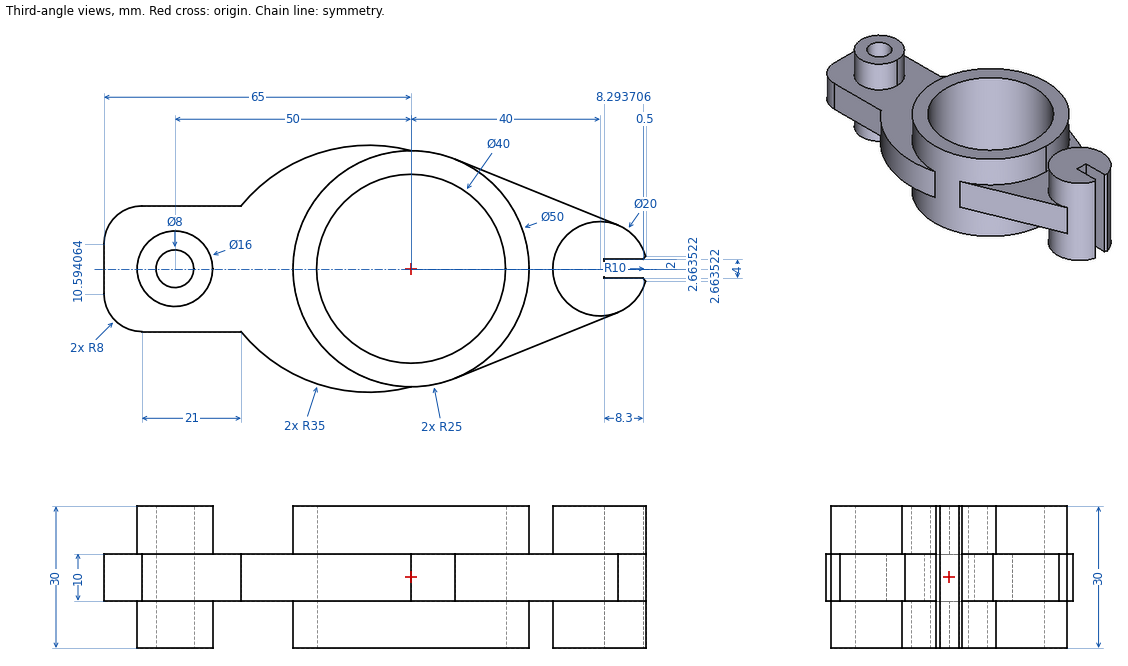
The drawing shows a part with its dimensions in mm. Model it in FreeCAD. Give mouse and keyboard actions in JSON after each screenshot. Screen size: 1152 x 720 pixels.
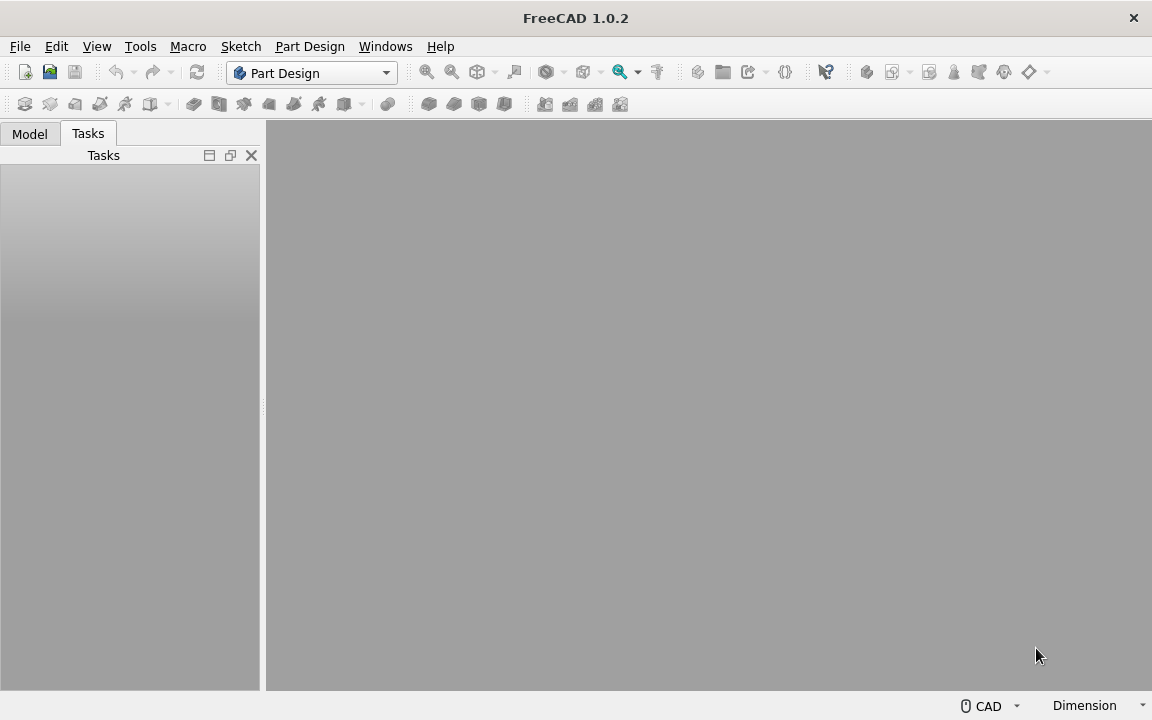
{"action": "left_click", "coordinate": [25, 72]}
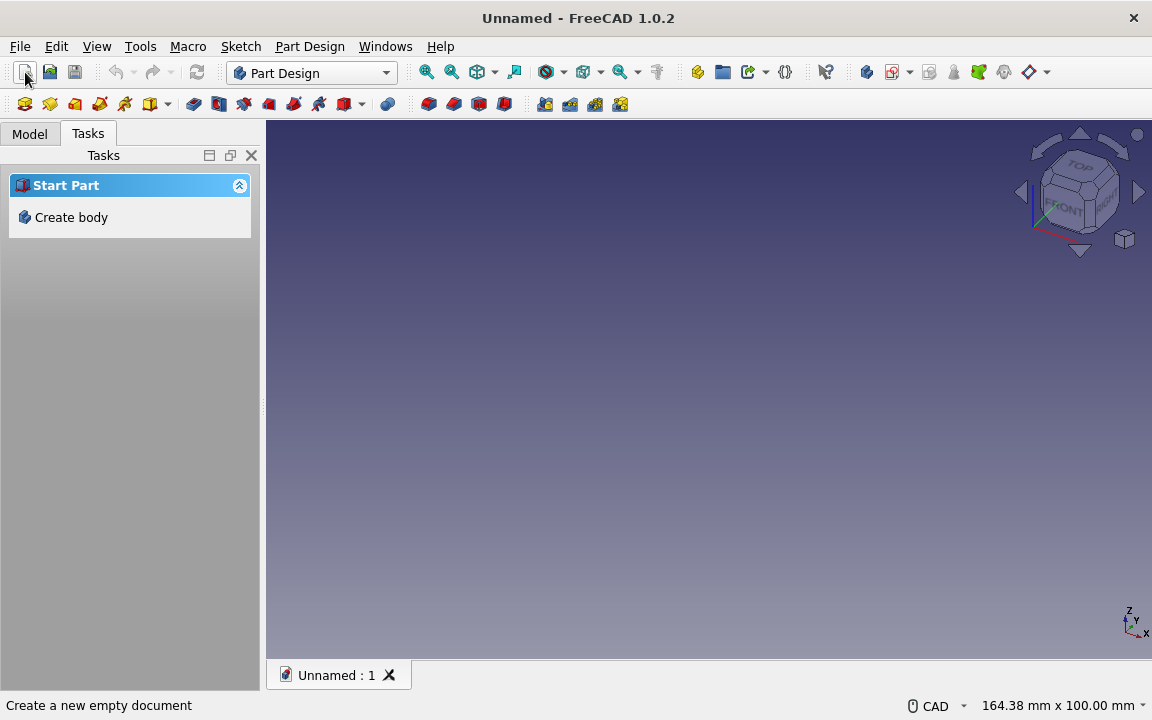
{"action": "left_click", "coordinate": [892, 72]}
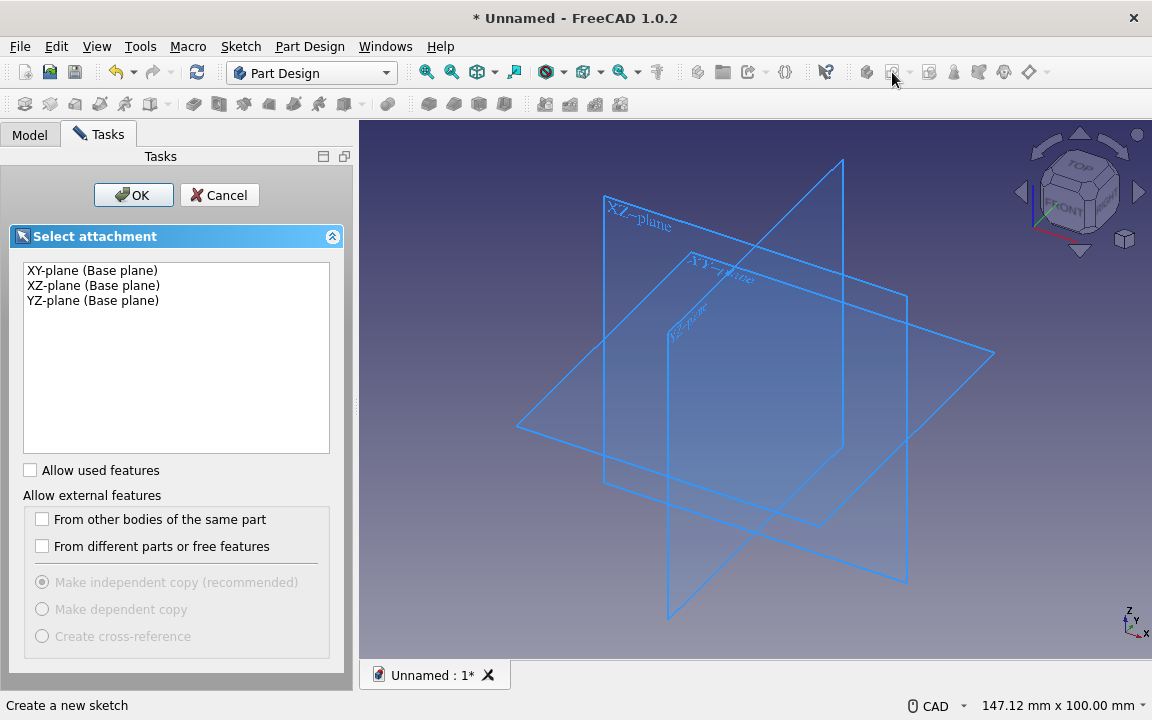
{"action": "left_click", "coordinate": [84, 270]}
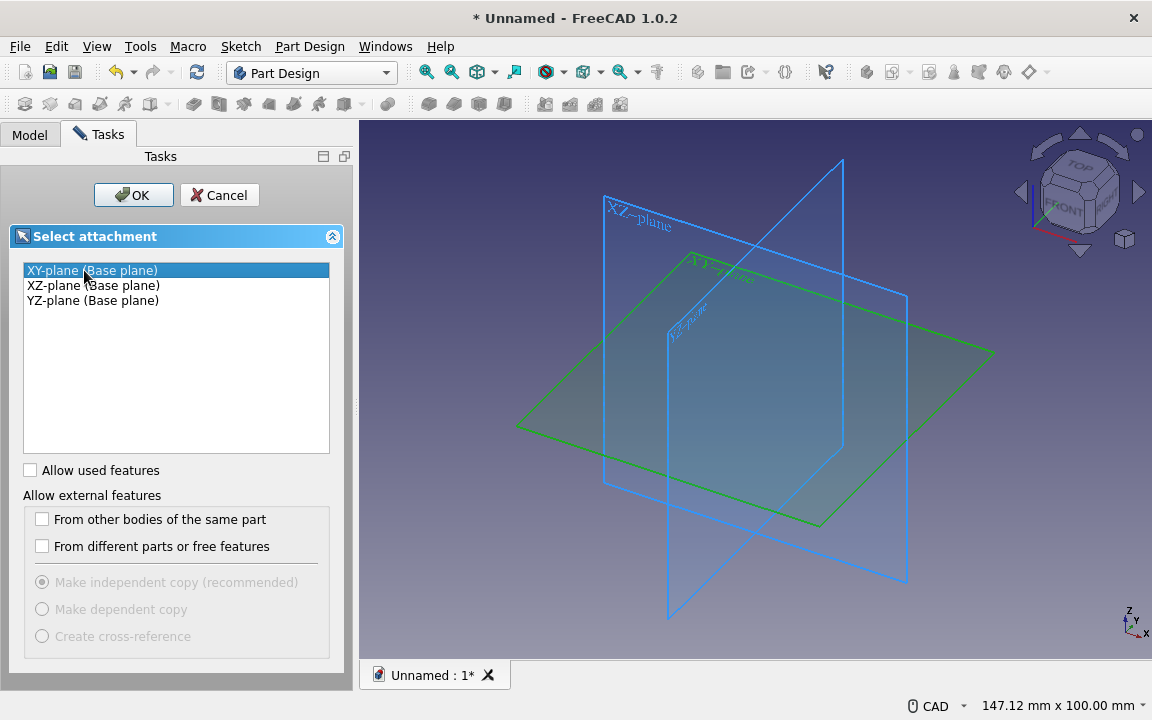
{"action": "left_click", "coordinate": [134, 195]}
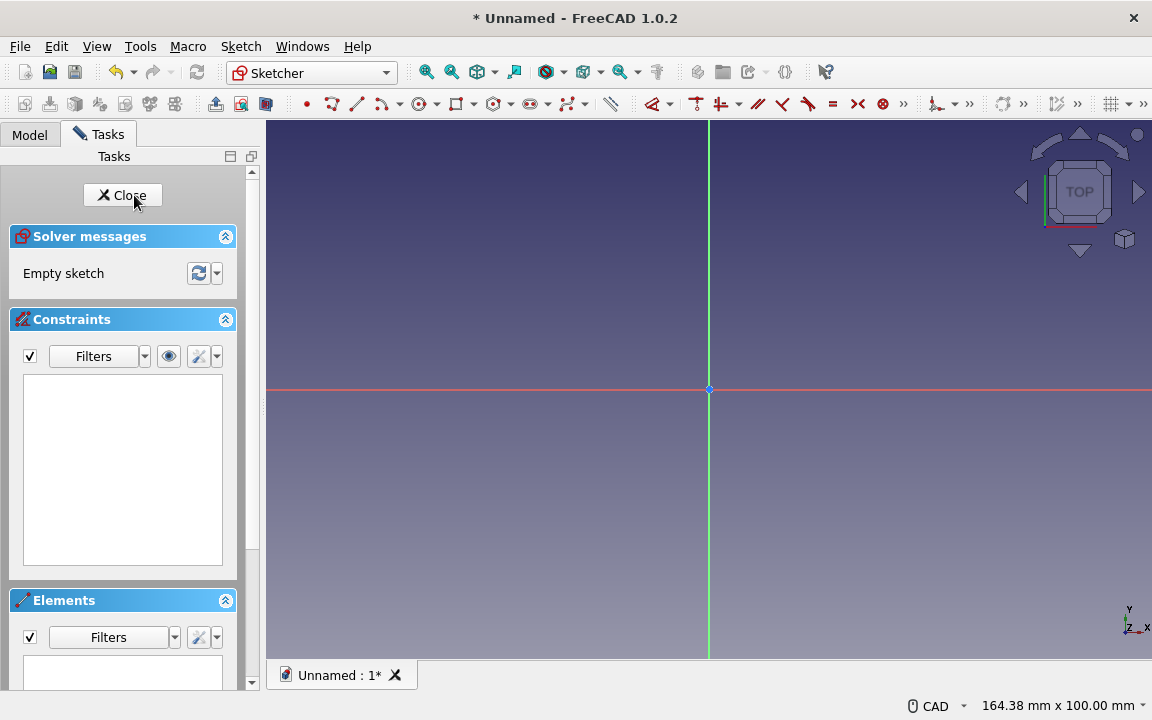
{"action": "left_click", "coordinate": [418, 104]}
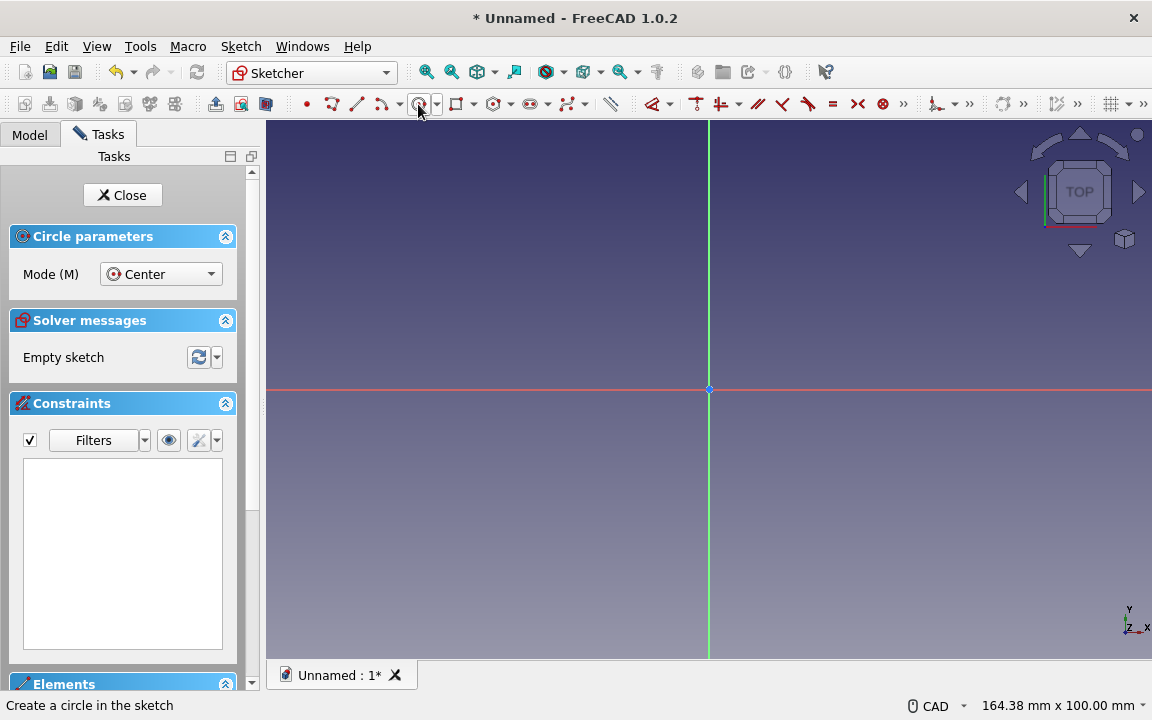
{"action": "left_click", "coordinate": [709, 390]}
{"action": "left_click", "coordinate": [804, 294]}
{"action": "key", "text": "Escape"}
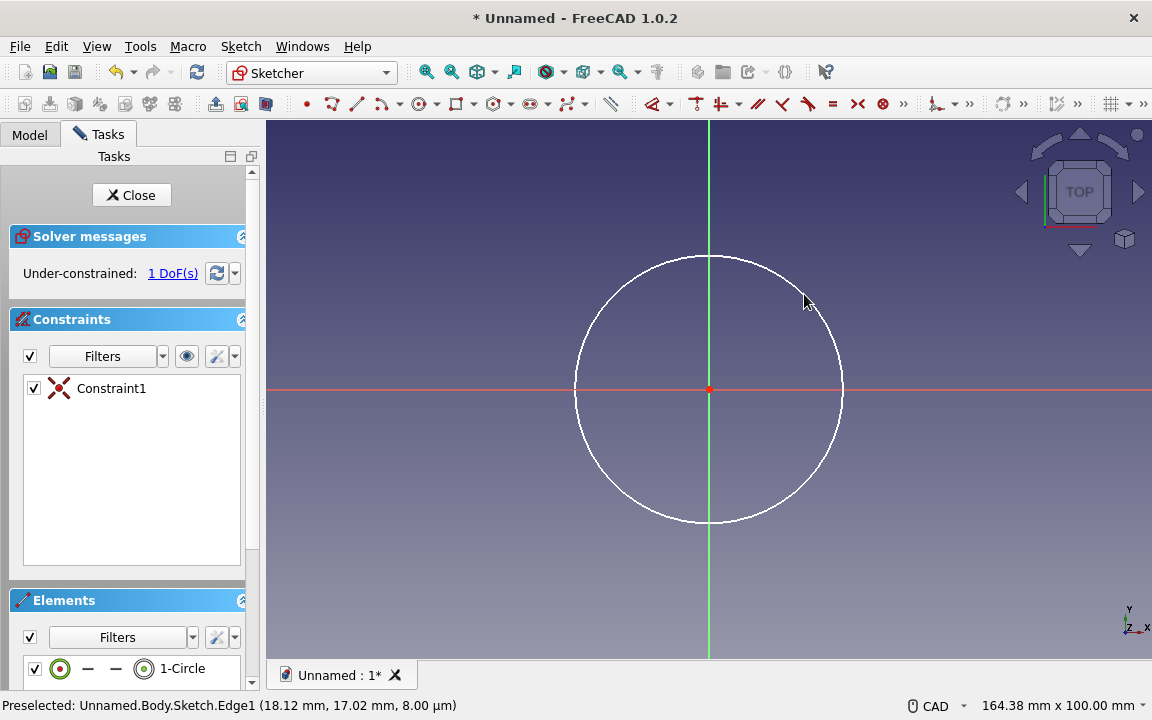
{"action": "left_click", "coordinate": [652, 104]}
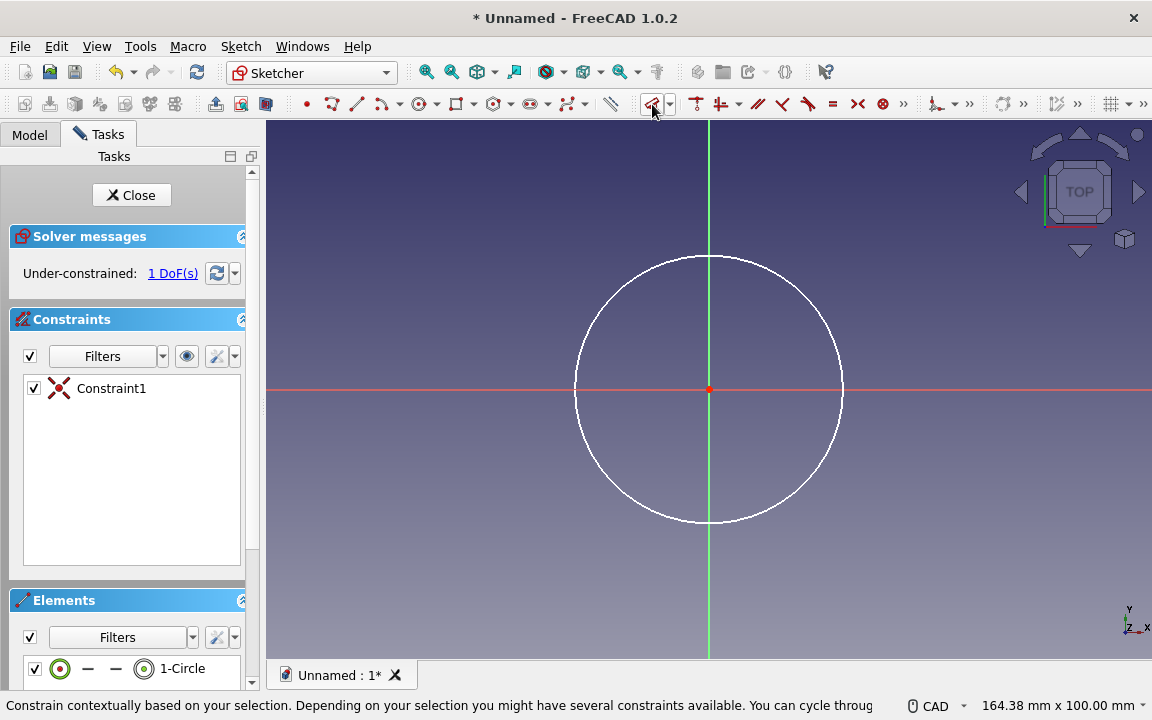
{"action": "left_click", "coordinate": [803, 294]}
{"action": "left_click", "coordinate": [825, 271]}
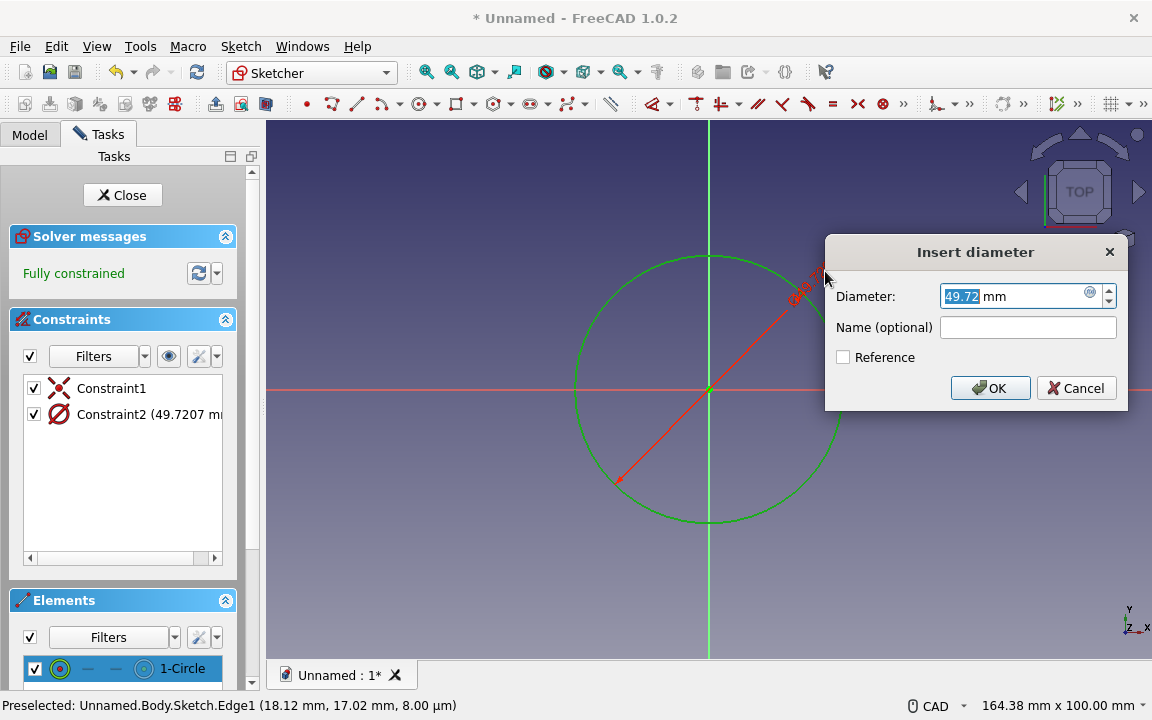
{"action": "type", "text": "50"}
{"action": "key", "text": "Return"}
{"action": "key", "text": "Escape"}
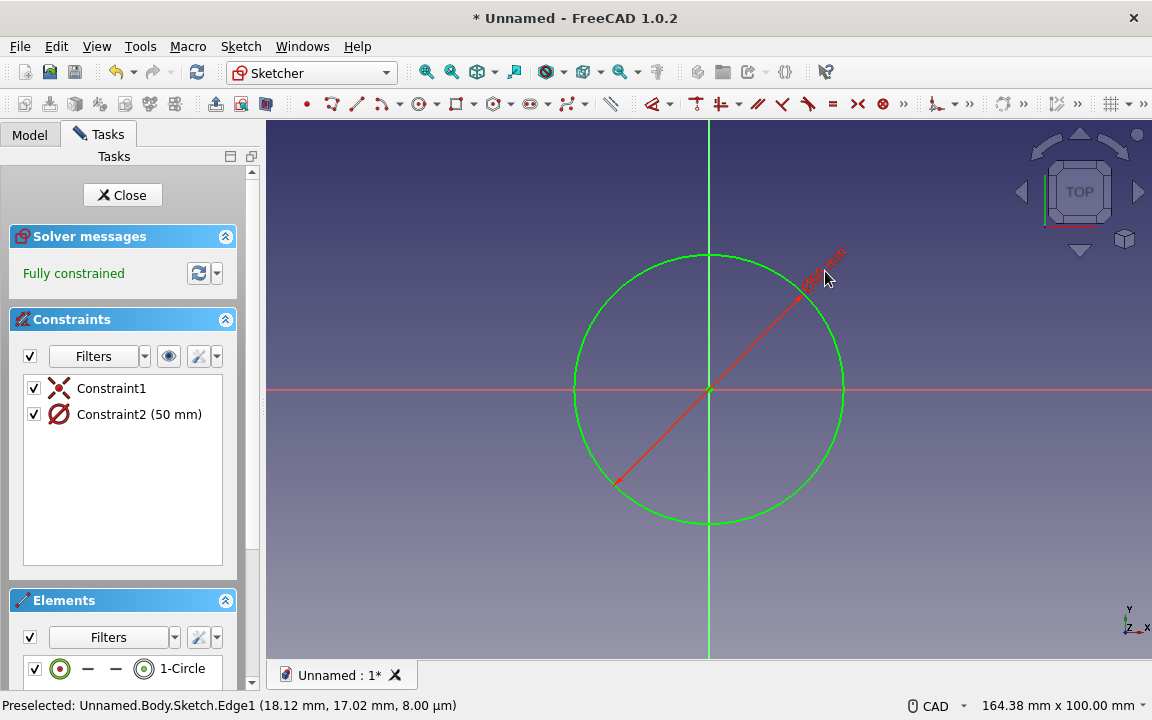
{"action": "left_click", "coordinate": [123, 195]}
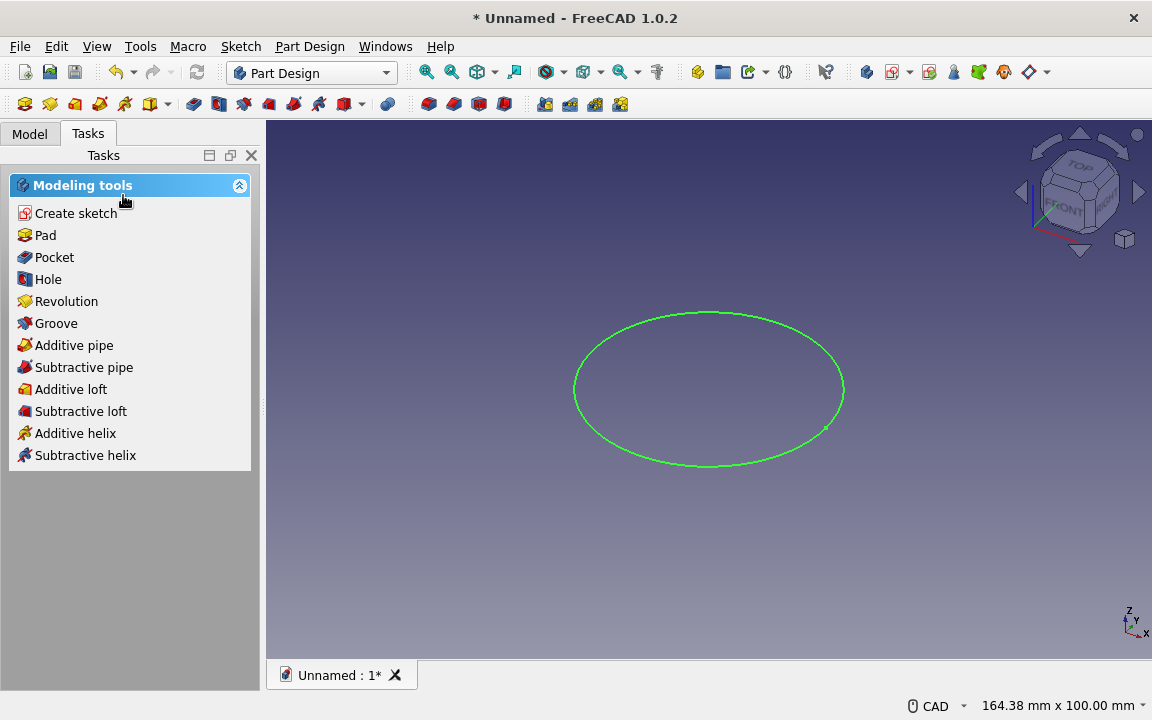
{"action": "left_click", "coordinate": [25, 104]}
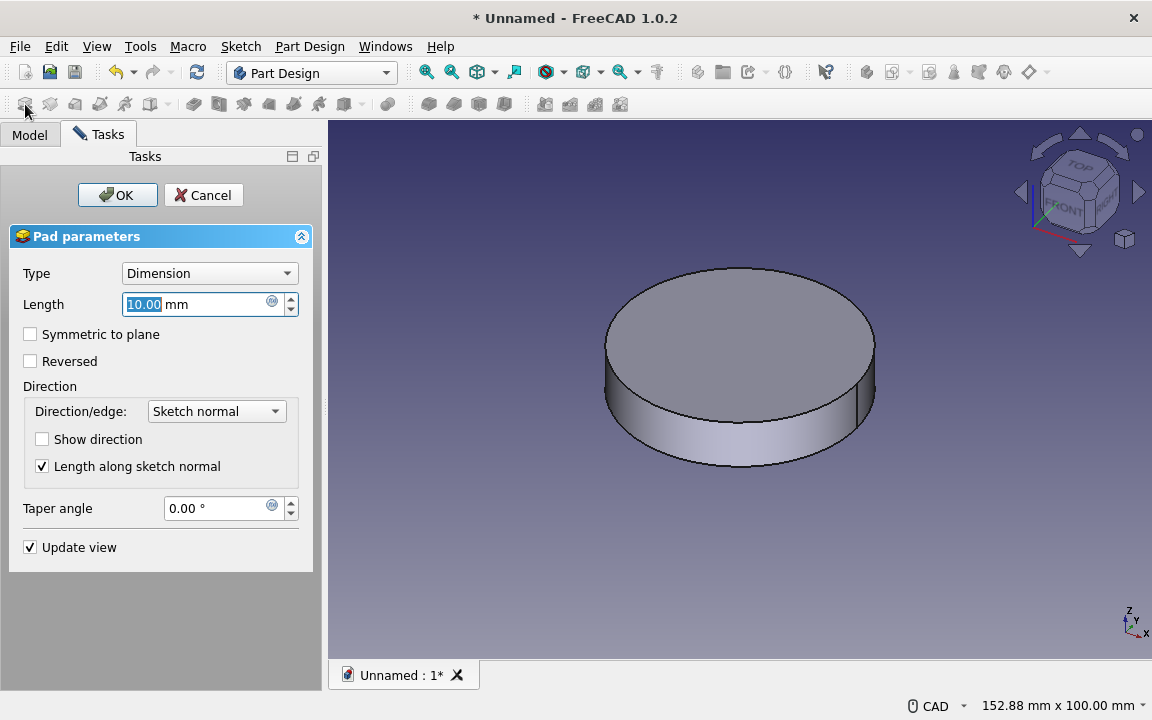
{"action": "type", "text": "30"}
{"action": "key", "text": "Tab"}